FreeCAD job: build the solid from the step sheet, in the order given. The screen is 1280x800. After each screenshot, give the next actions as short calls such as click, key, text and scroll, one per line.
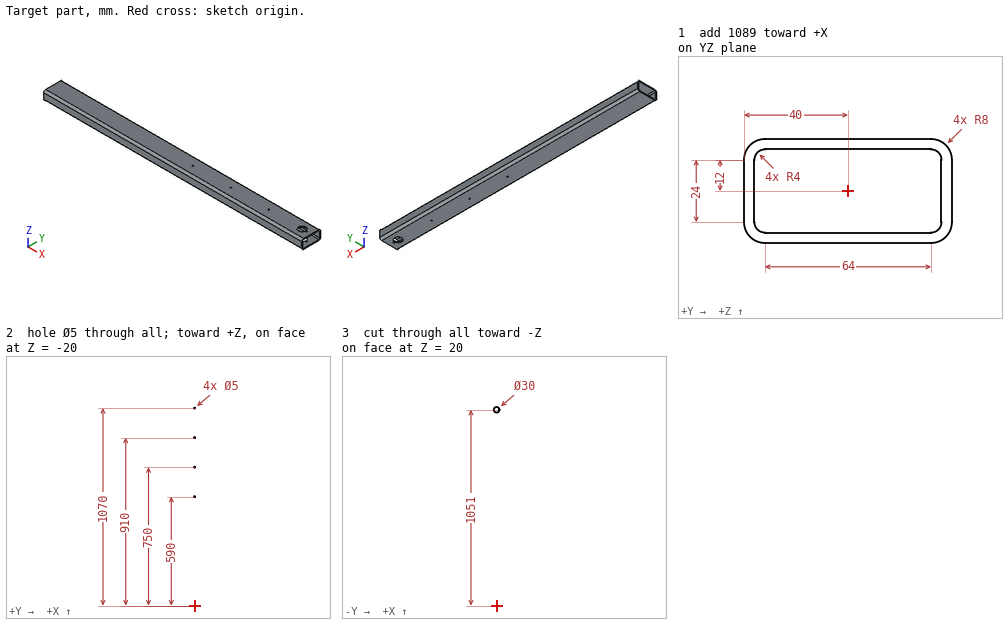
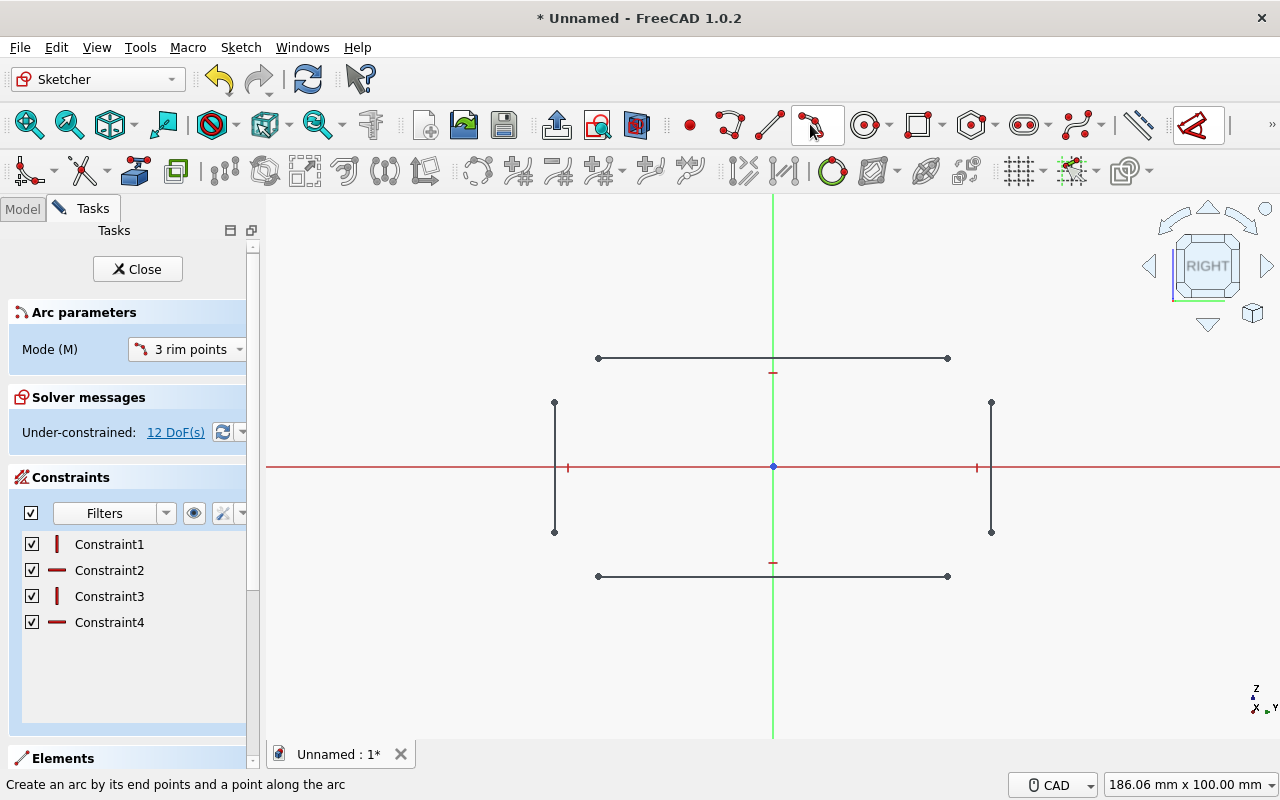
click(555, 533)
click(599, 577)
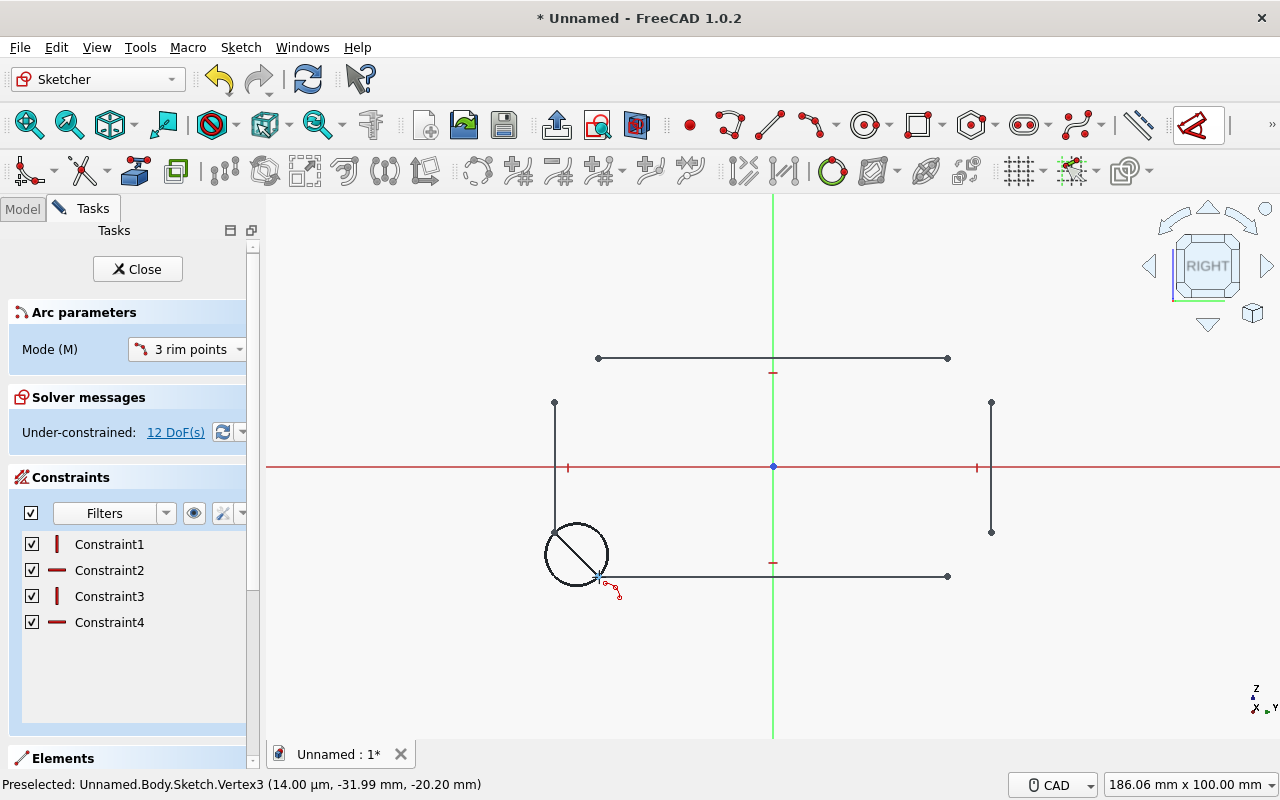
scroll(568, 563, up, 2)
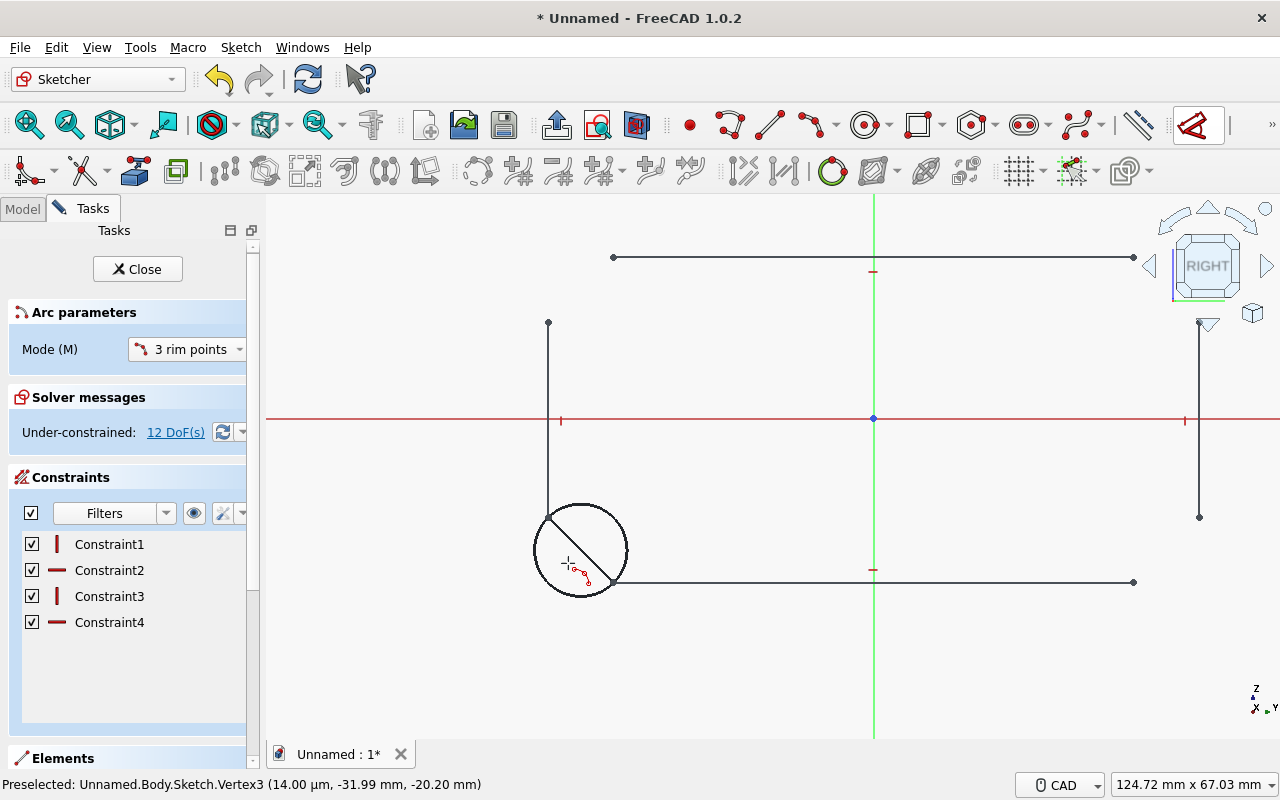
click(568, 562)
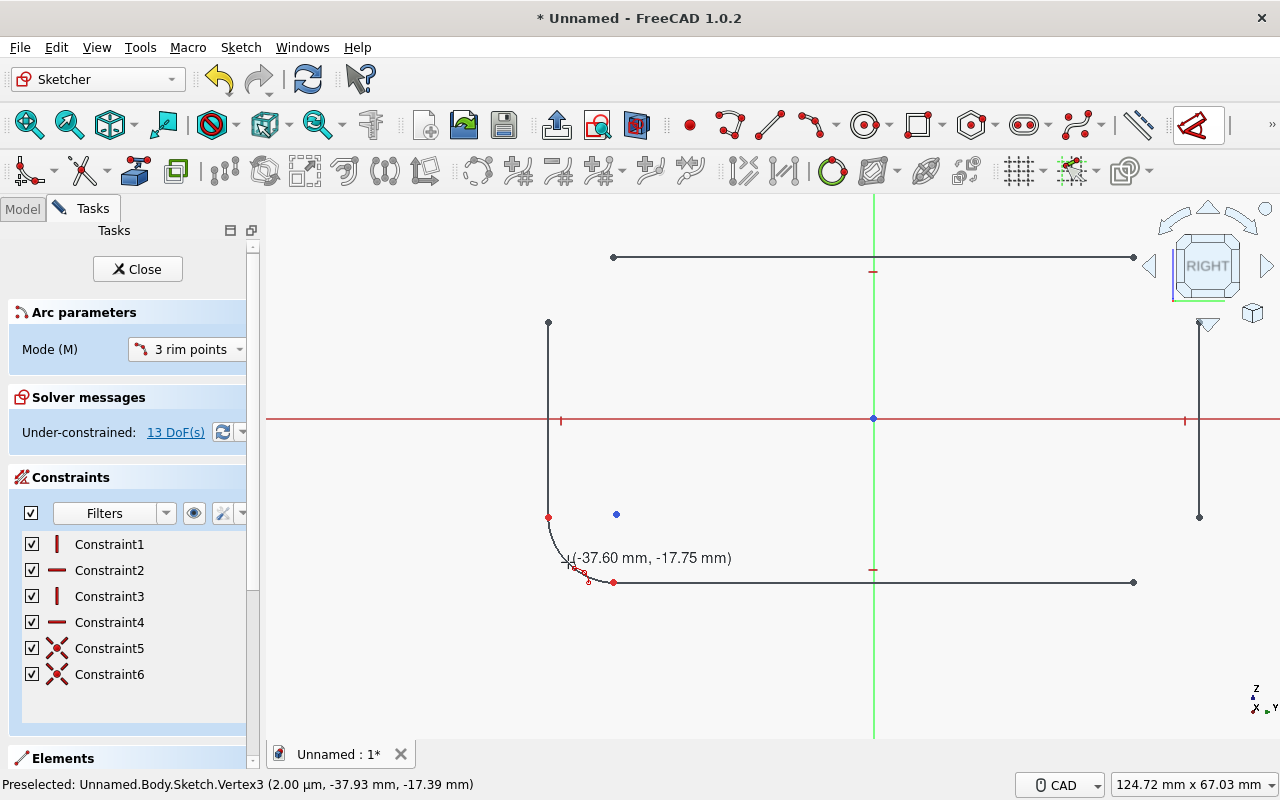
scroll(294, 682, down, 1)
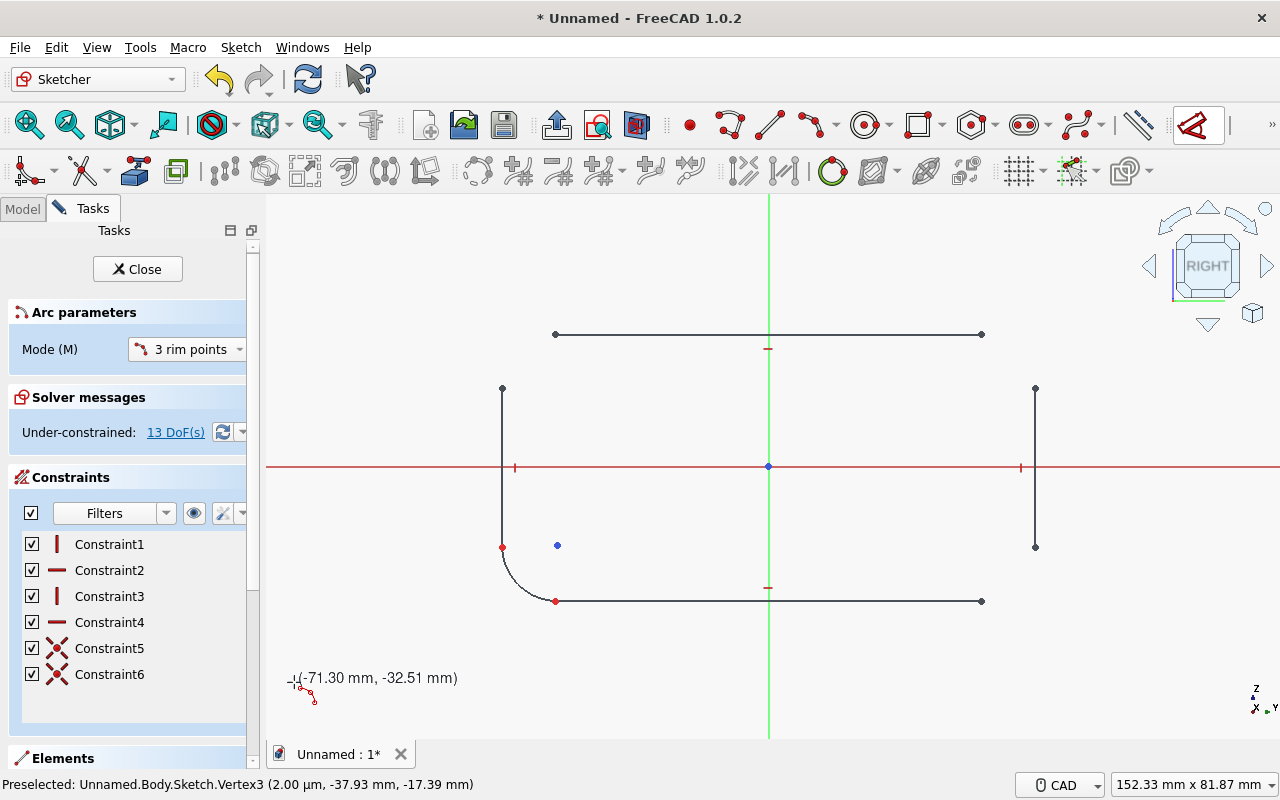
click(982, 601)
click(1035, 548)
click(1019, 584)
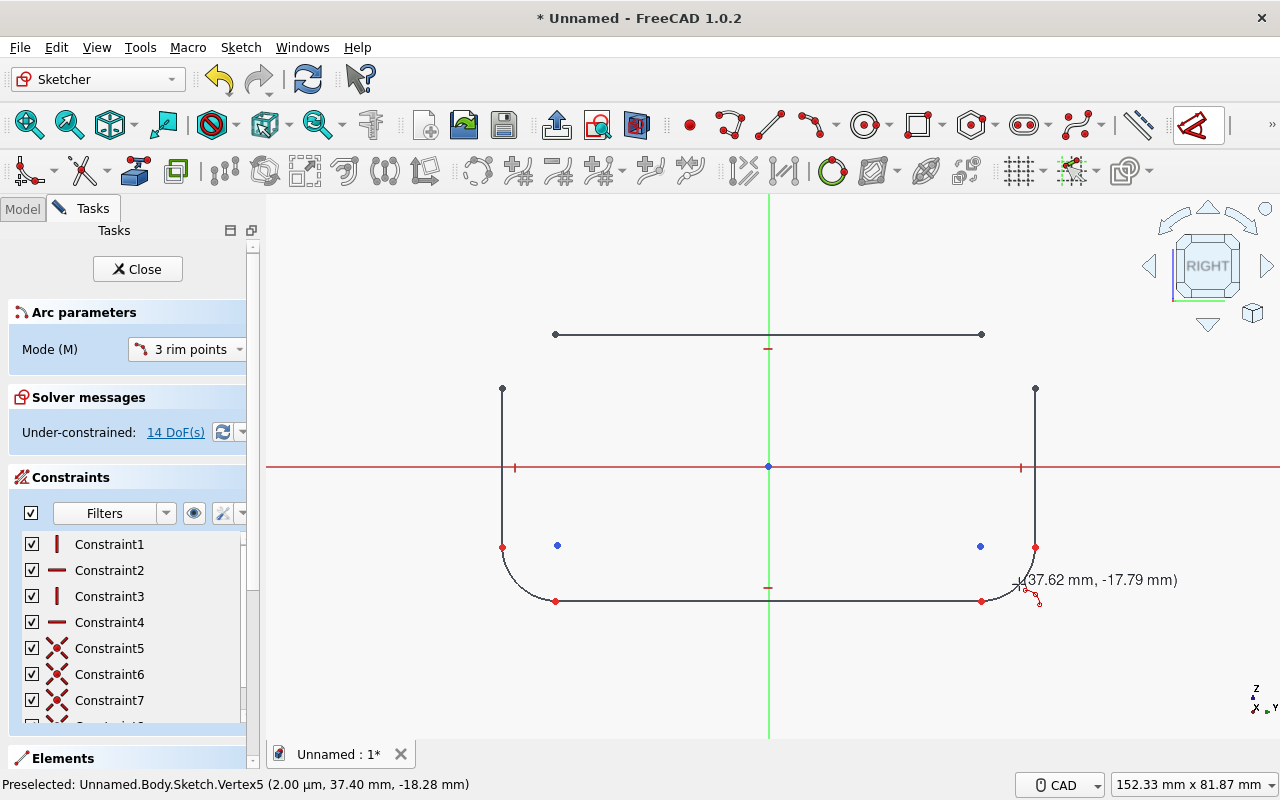
click(1035, 388)
click(982, 335)
click(1019, 349)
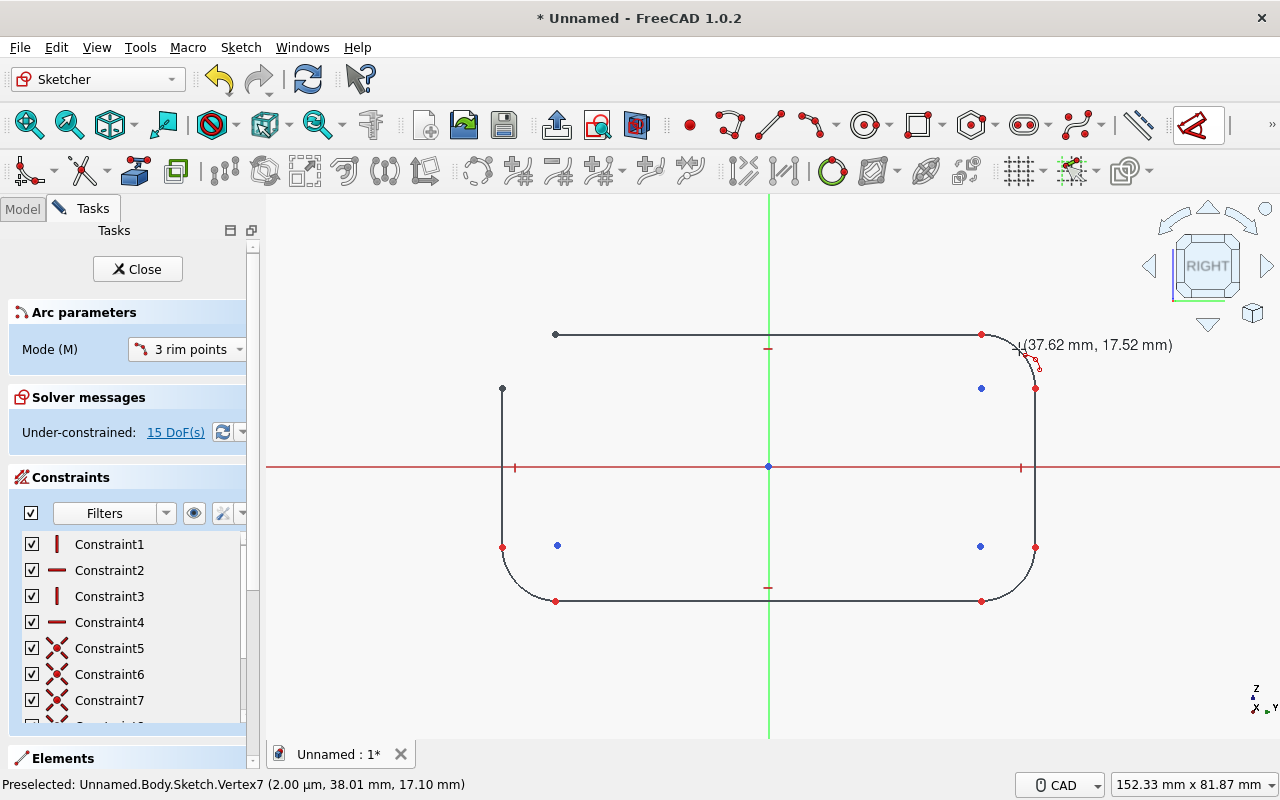
click(556, 335)
click(502, 388)
click(518, 349)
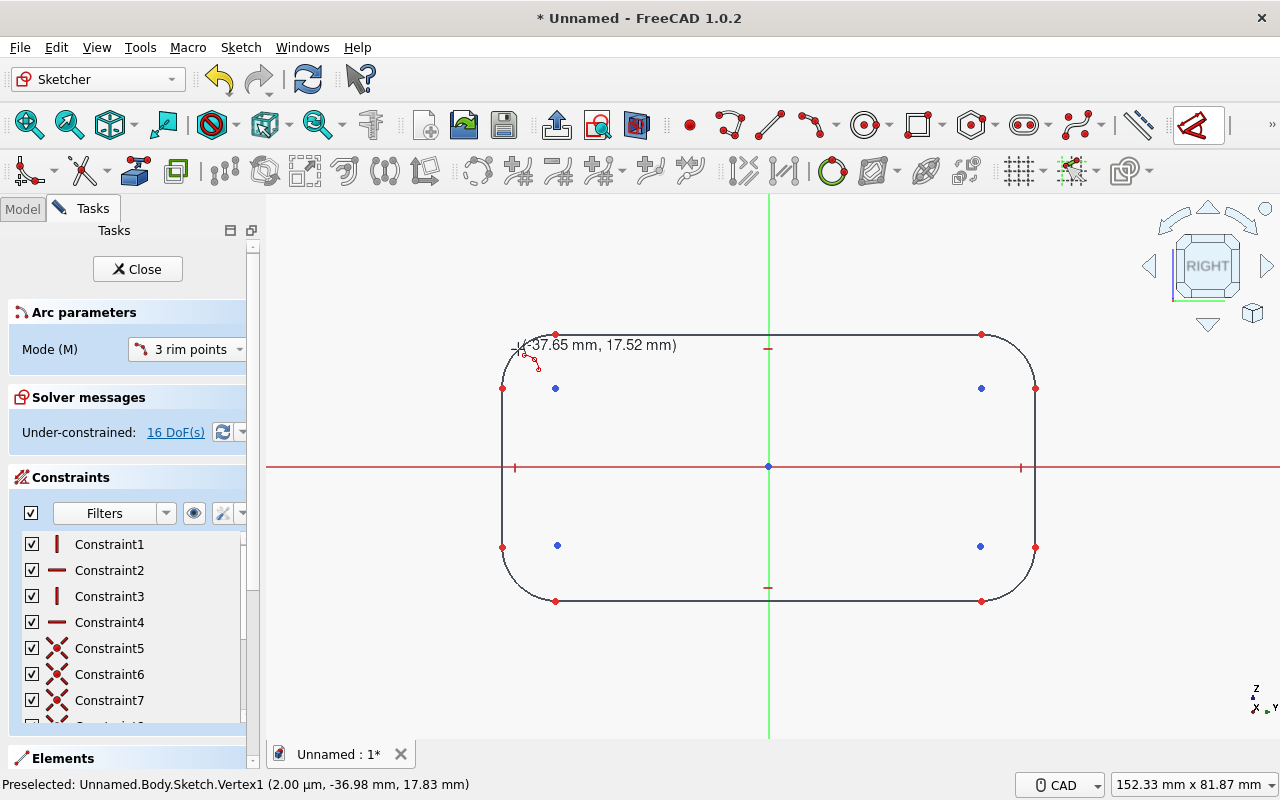
click(770, 126)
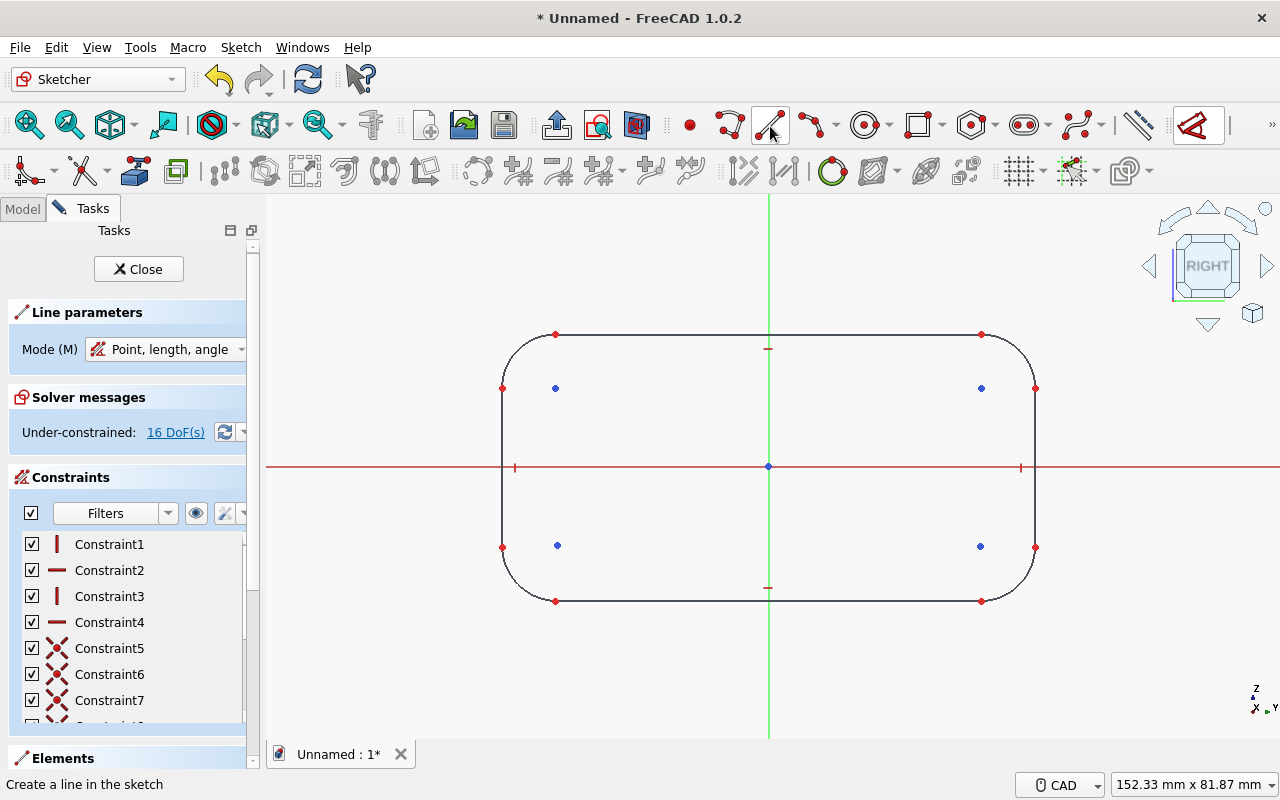
click(529, 546)
click(529, 387)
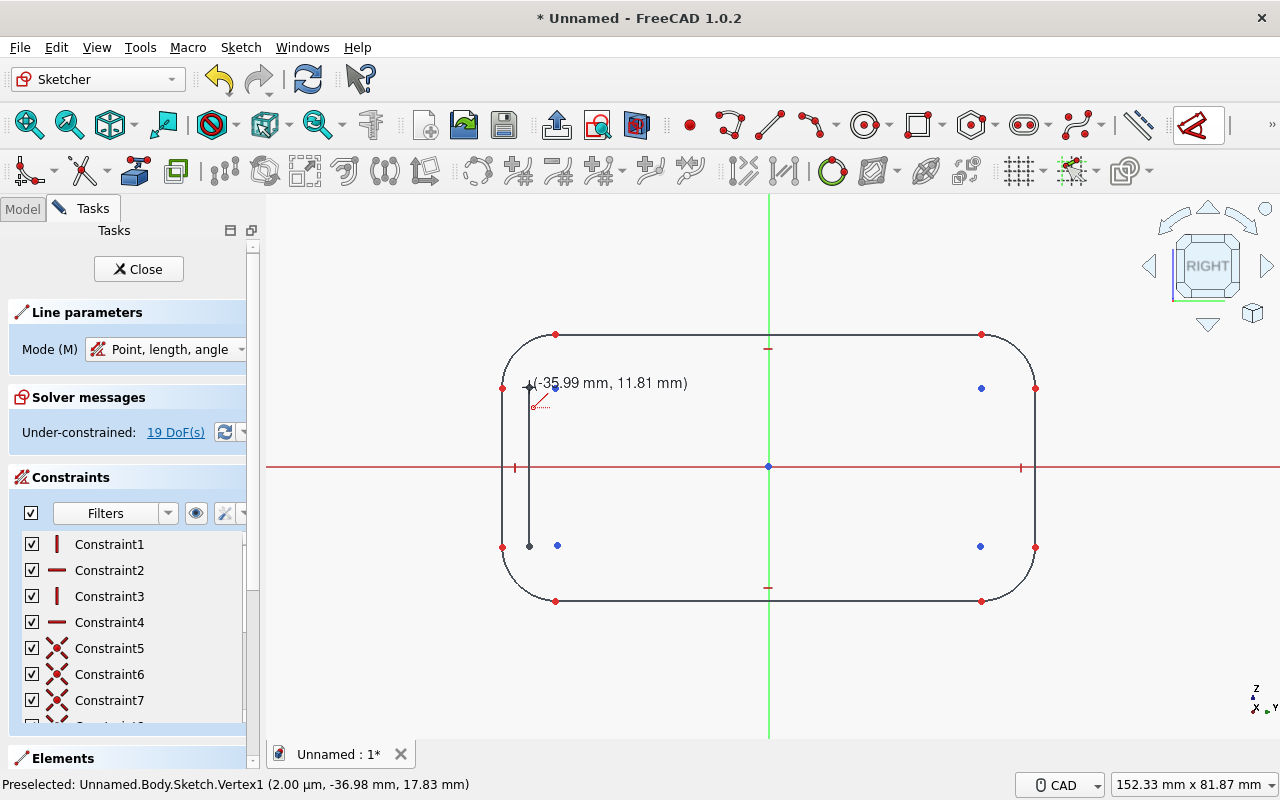
click(556, 360)
click(982, 360)